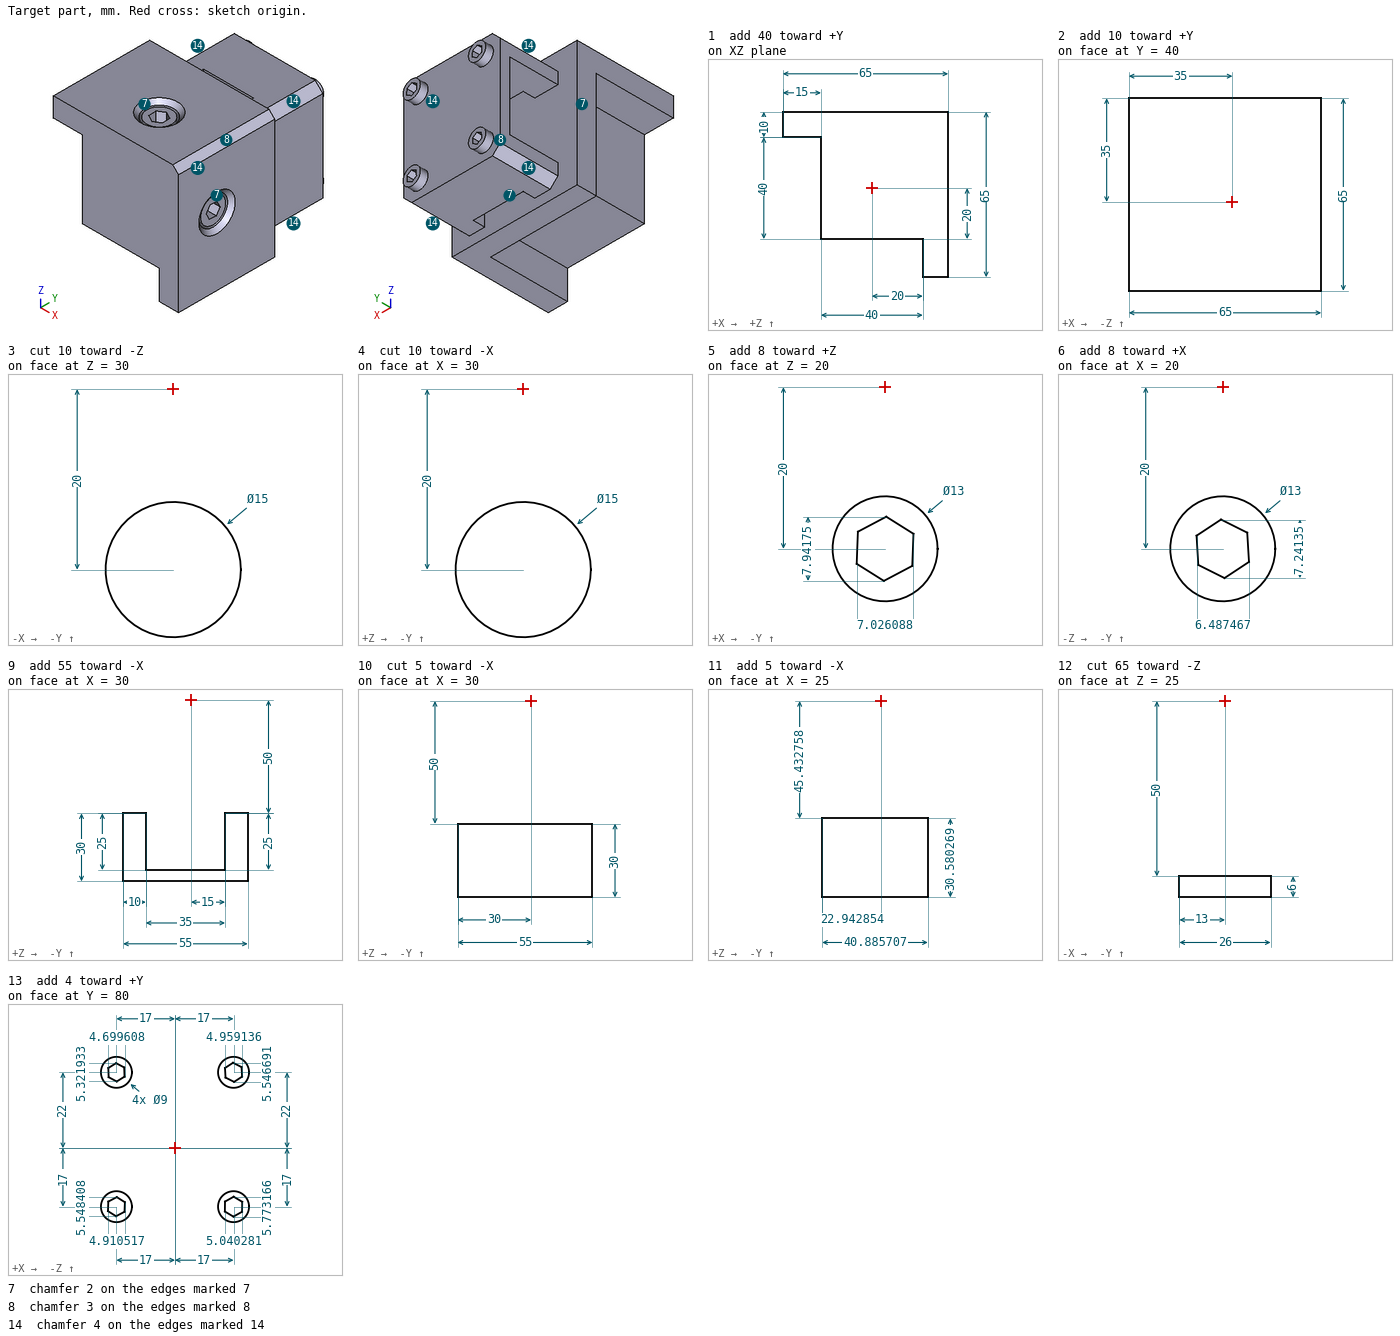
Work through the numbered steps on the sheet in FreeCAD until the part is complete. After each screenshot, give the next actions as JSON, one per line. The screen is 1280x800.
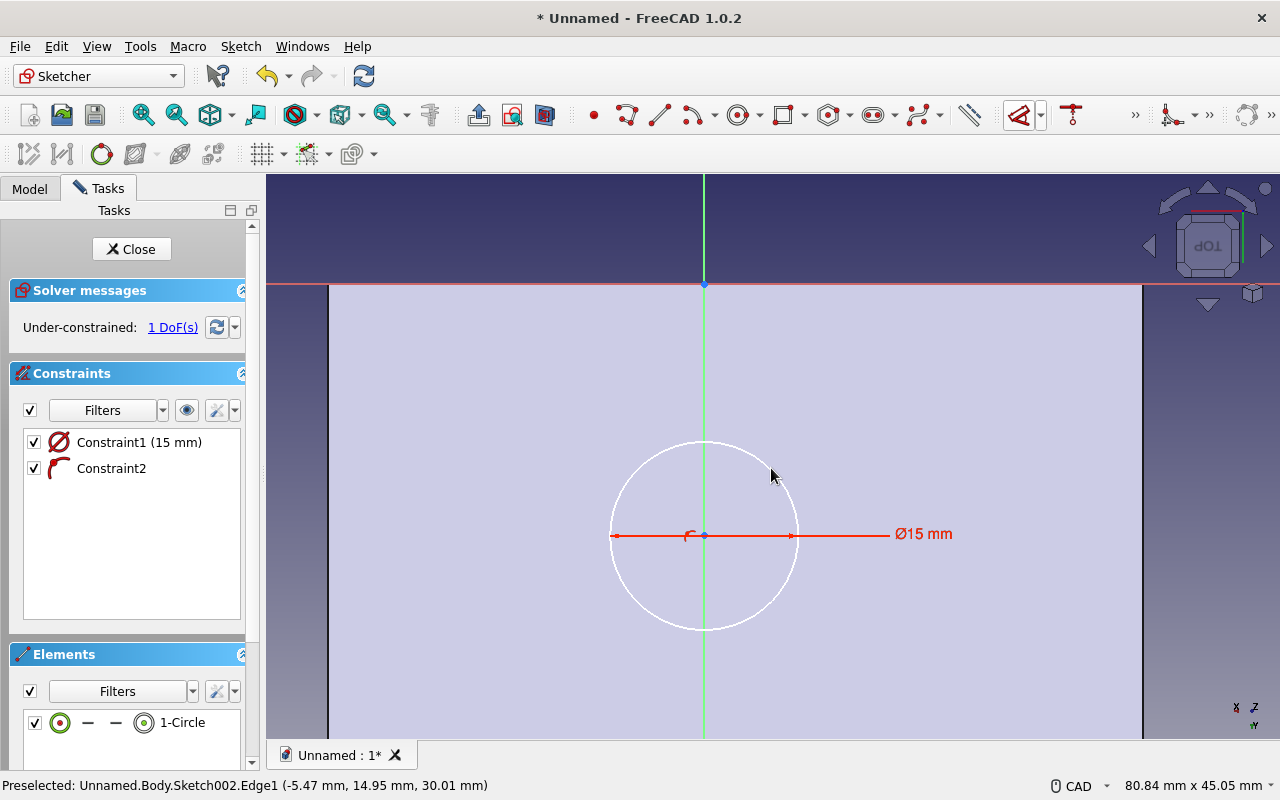
{"action": "left_click", "coordinate": [704, 536]}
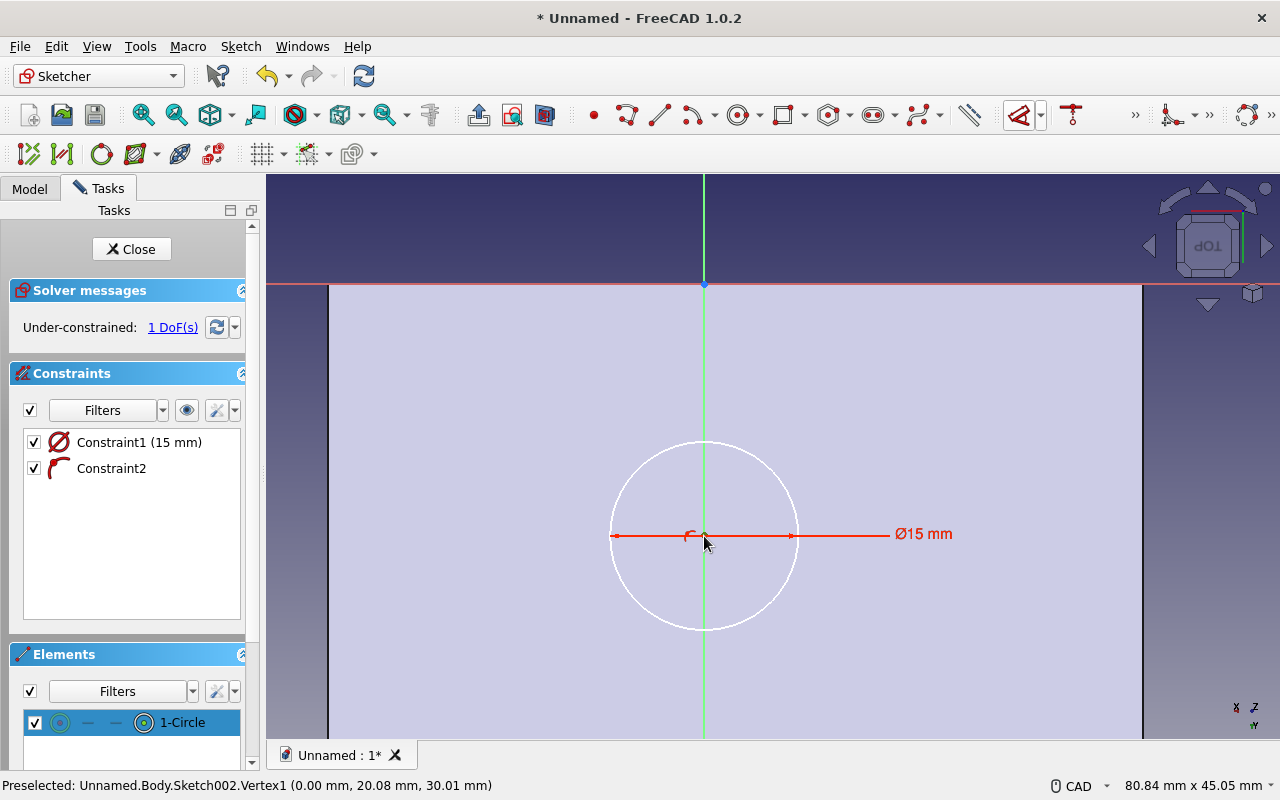
{"action": "left_click", "coordinate": [1040, 116]}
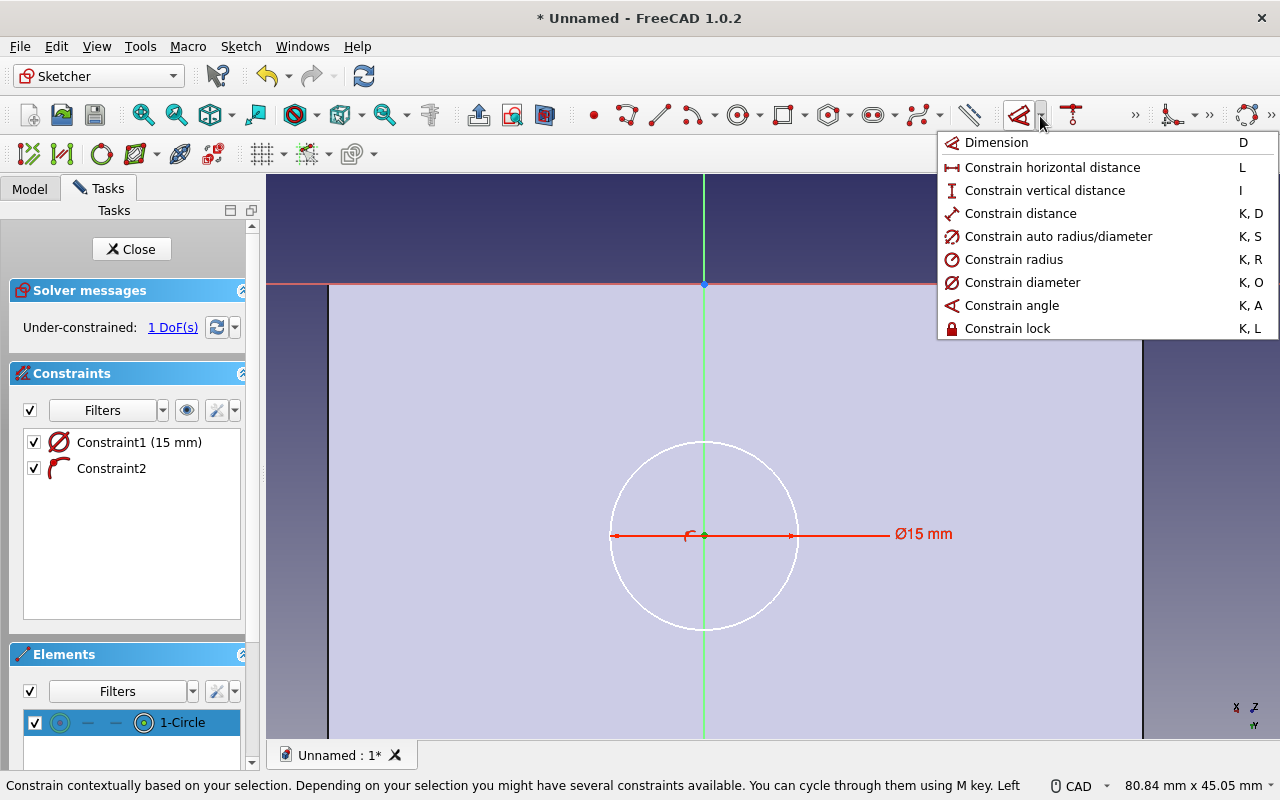
{"action": "left_click", "coordinate": [1108, 190]}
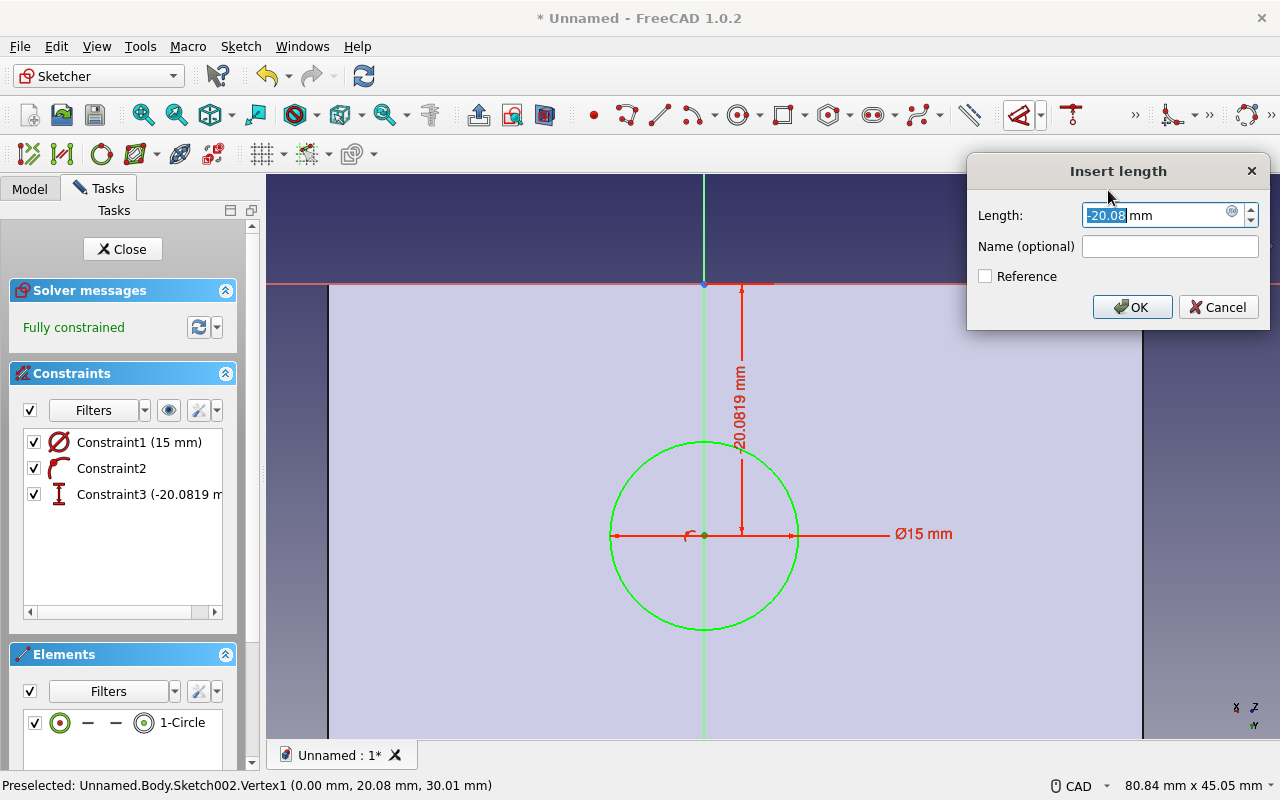
{"action": "type", "text": "-20"}
{"action": "key", "text": "Return"}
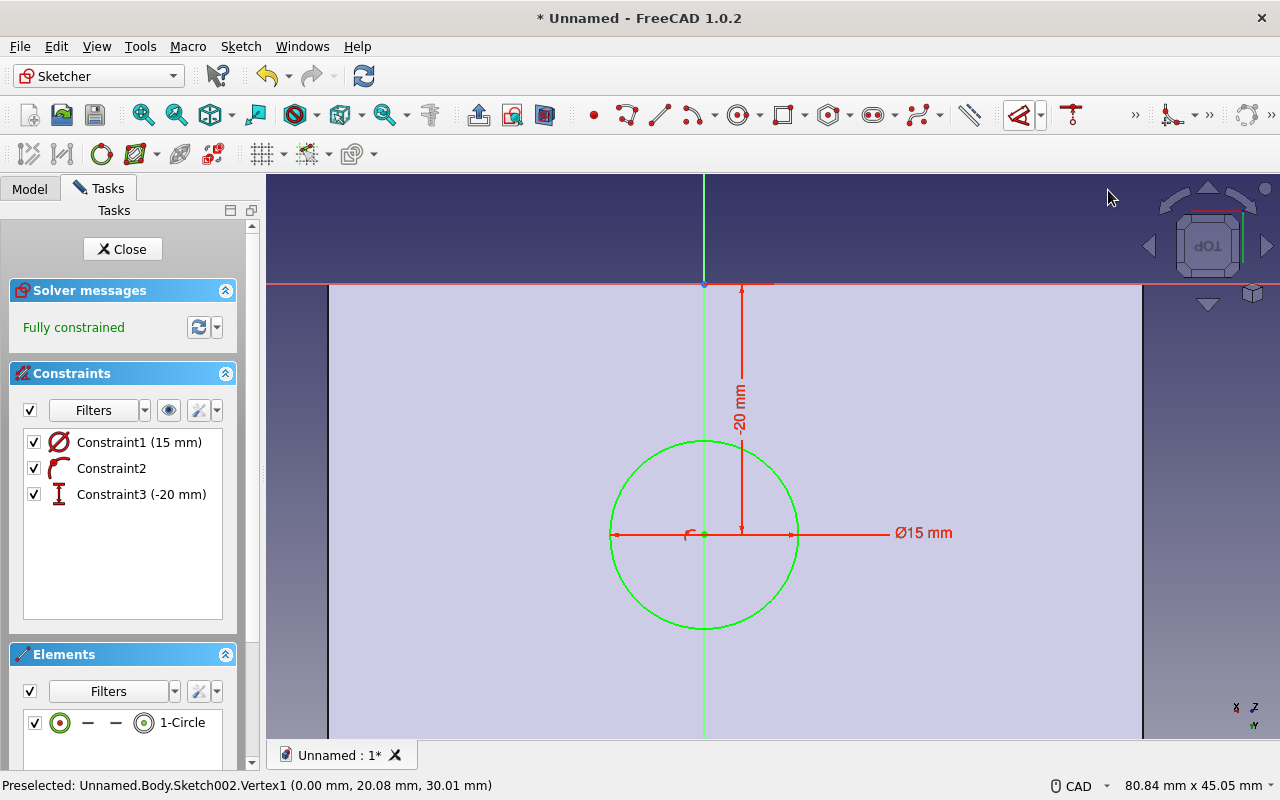
{"action": "left_click", "coordinate": [123, 249]}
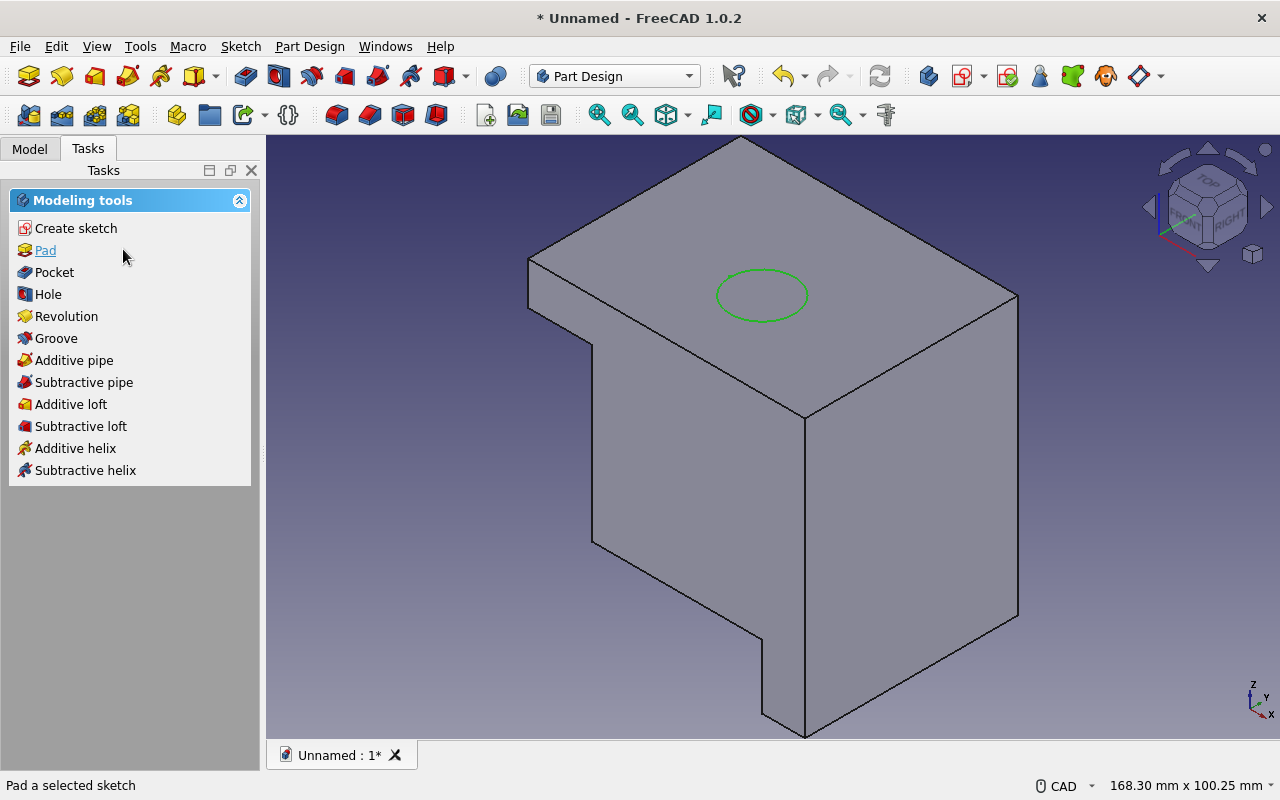
{"action": "left_click", "coordinate": [246, 76]}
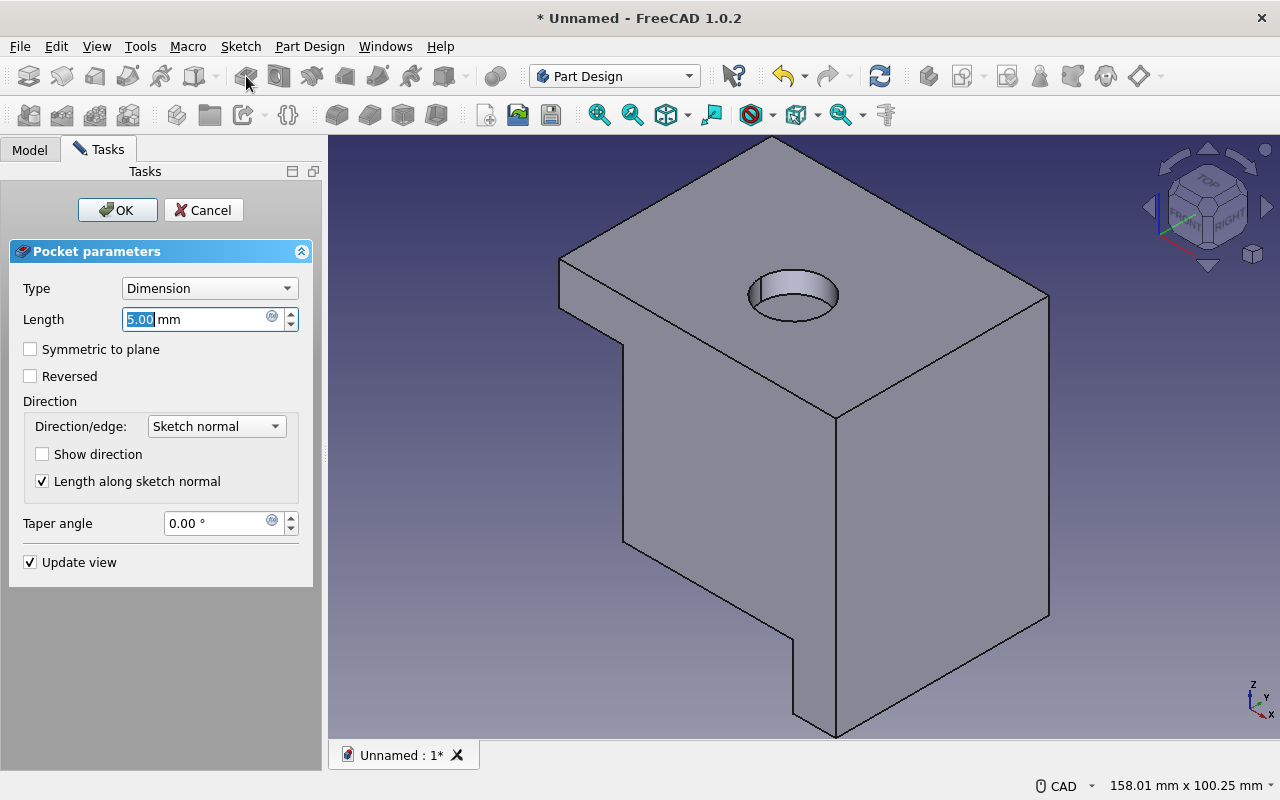
{"action": "type", "text": "10"}
{"action": "key", "text": "Tab"}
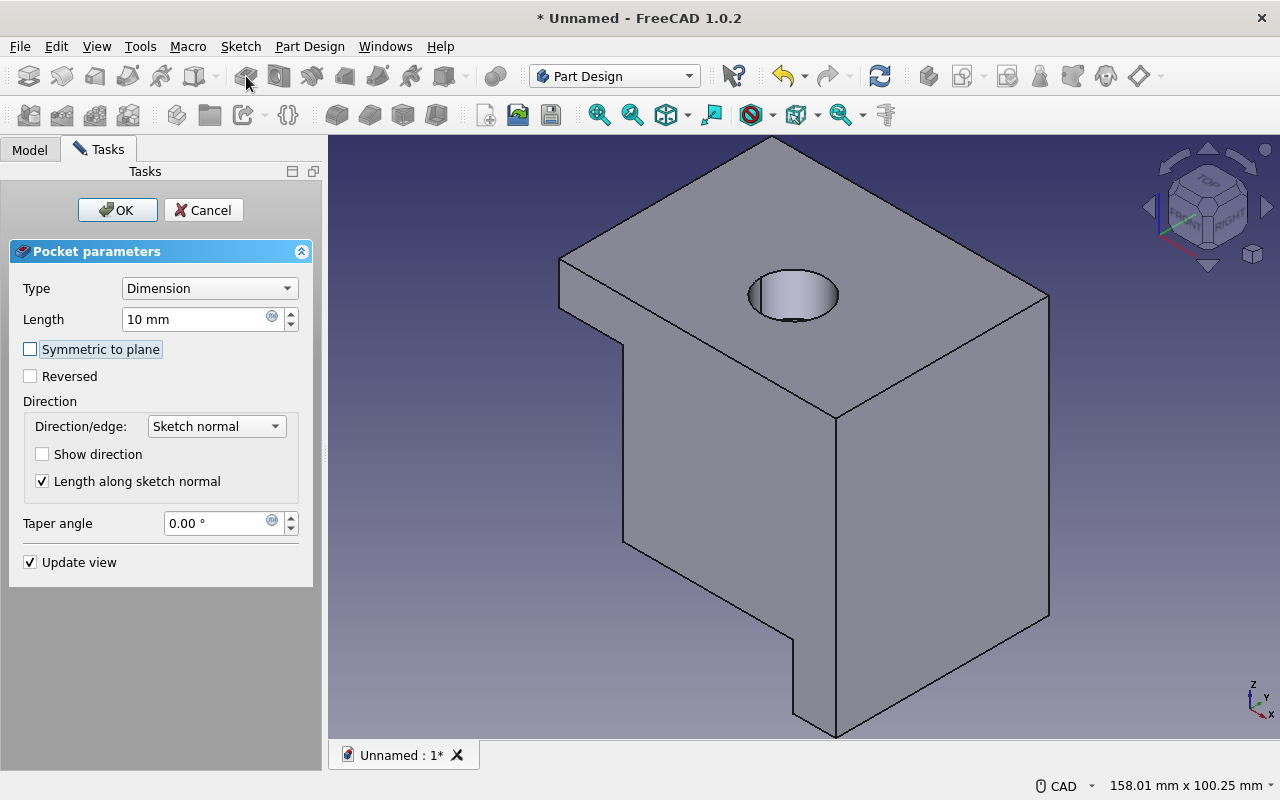
{"action": "left_click", "coordinate": [118, 210]}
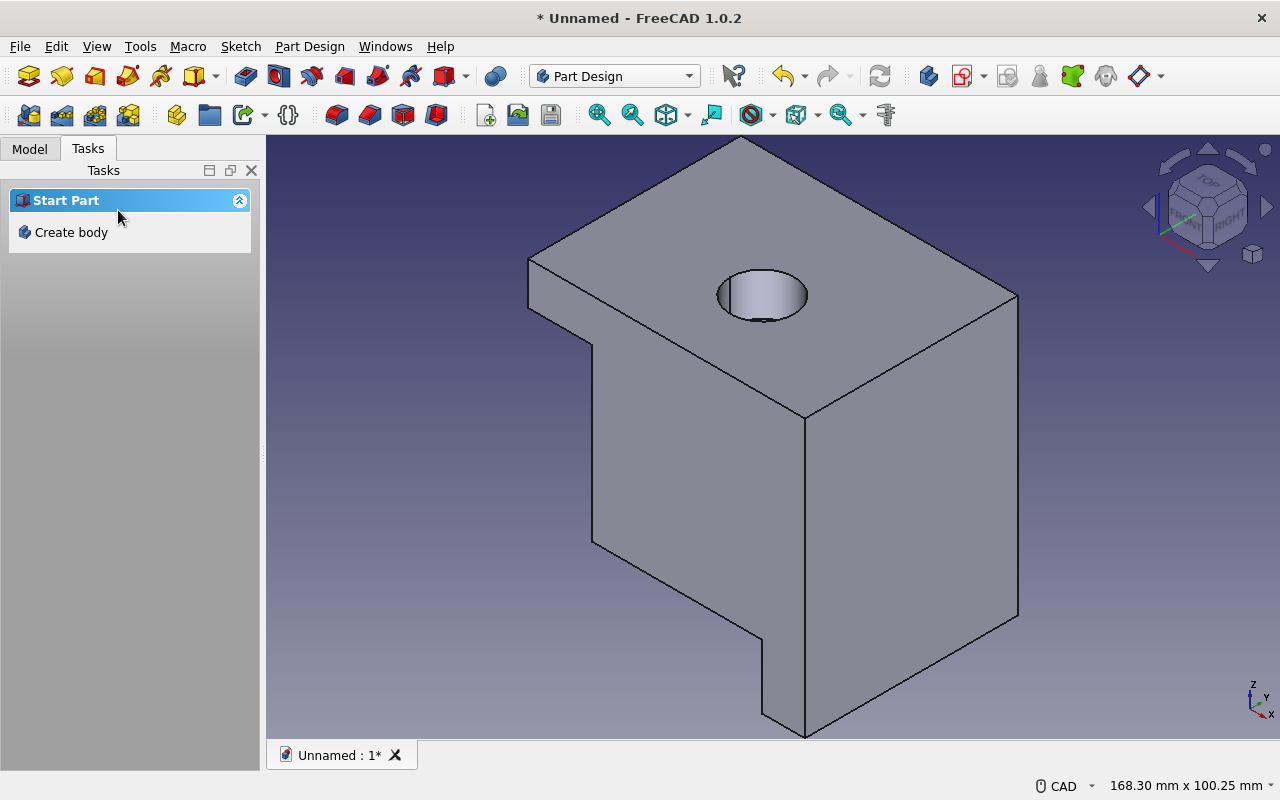
{"action": "left_click", "coordinate": [911, 516]}